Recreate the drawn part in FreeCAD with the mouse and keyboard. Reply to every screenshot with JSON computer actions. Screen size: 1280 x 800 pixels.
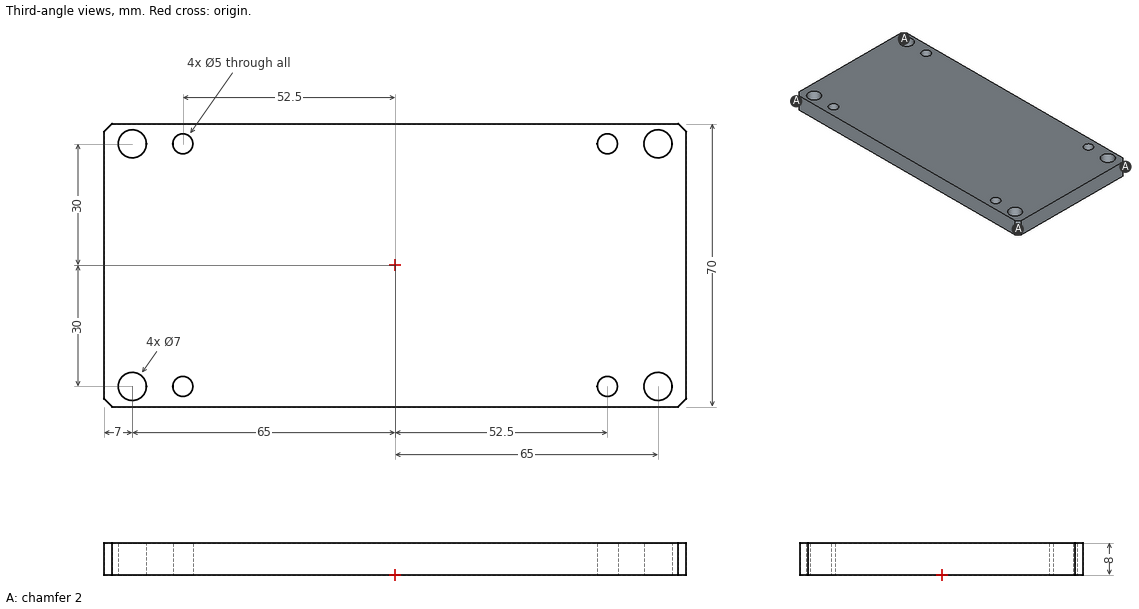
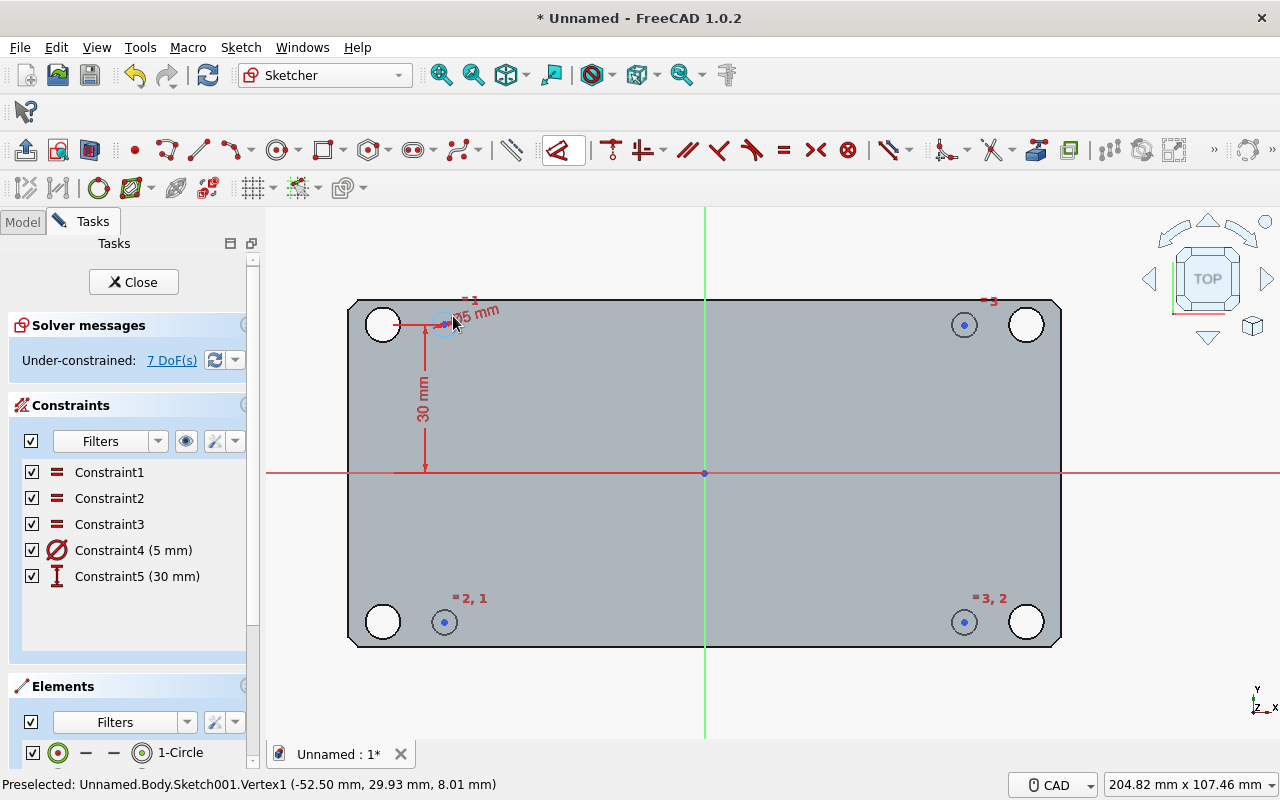
{"action": "left_click", "coordinate": [445, 622]}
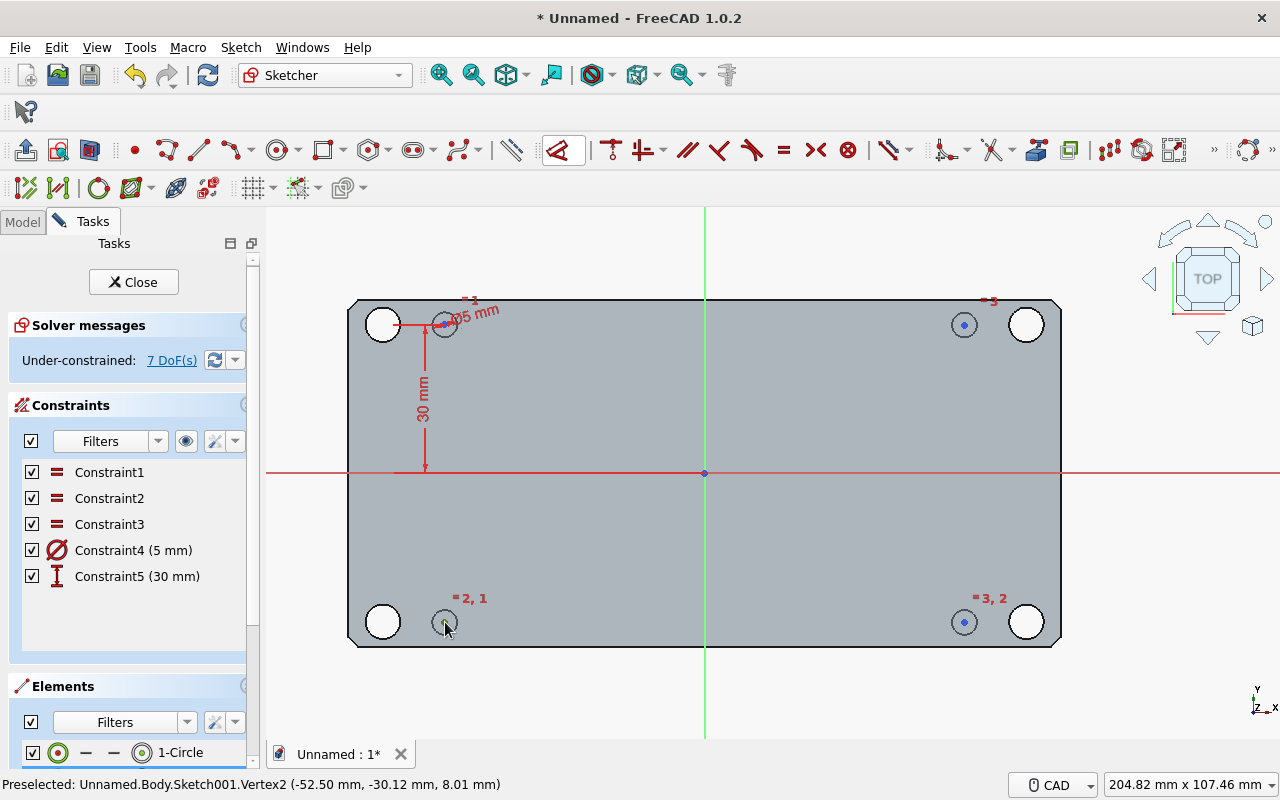
{"action": "key", "text": "i"}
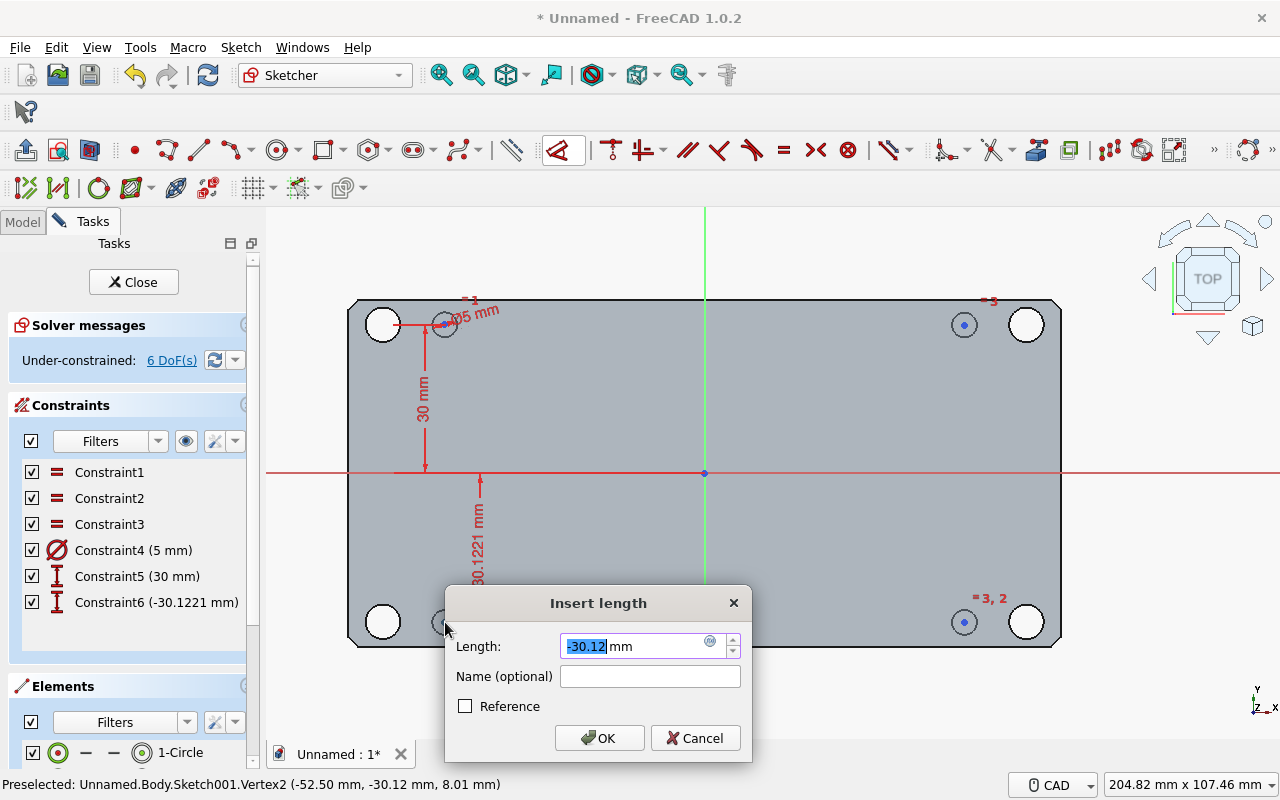
{"action": "type", "text": "-30"}
{"action": "key", "text": "Return"}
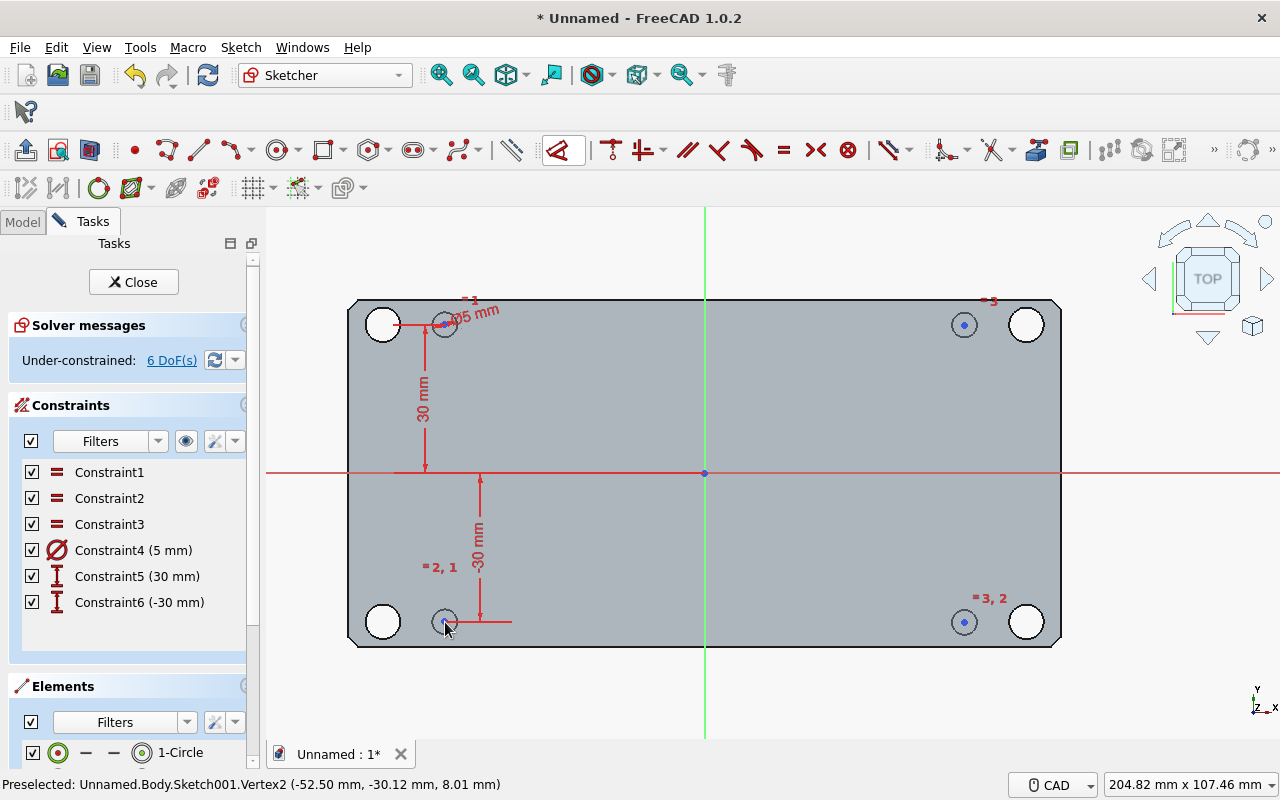
{"action": "left_click", "coordinate": [964, 622]}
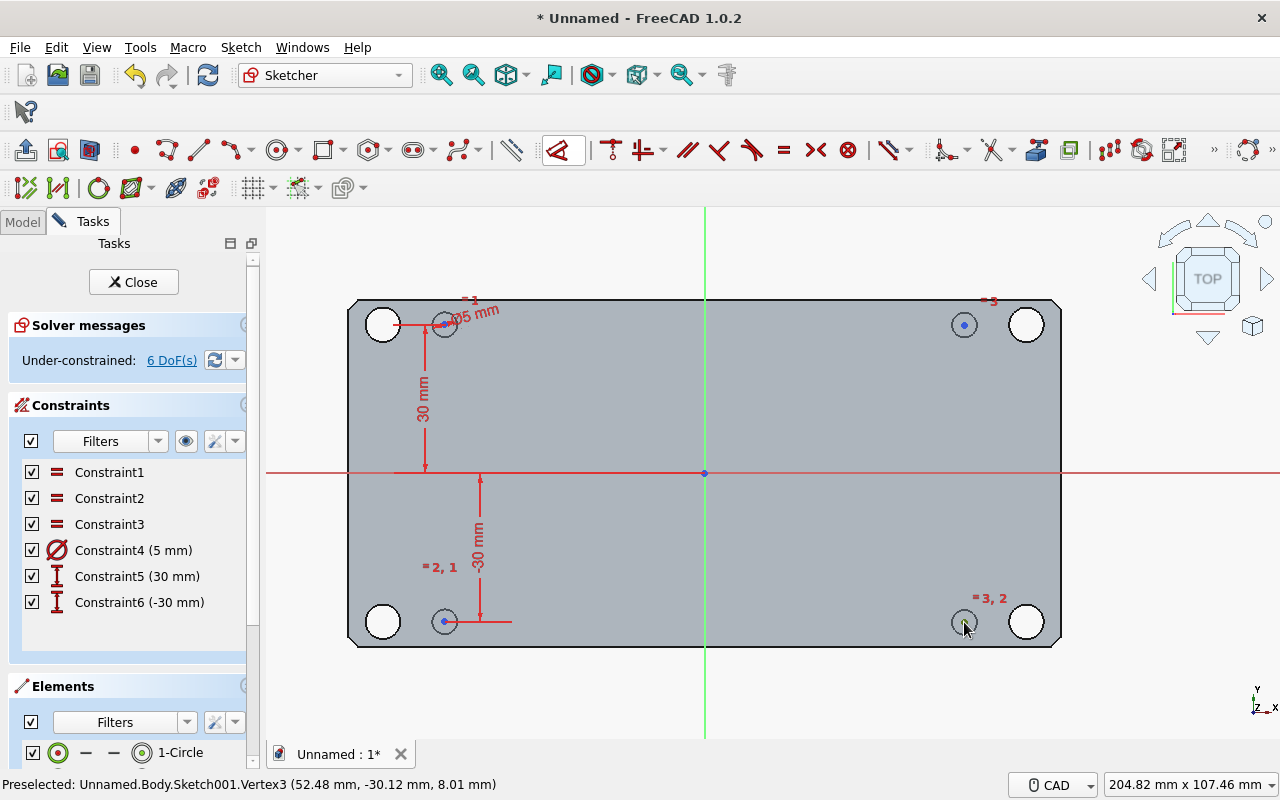
{"action": "left_click", "coordinate": [580, 150]}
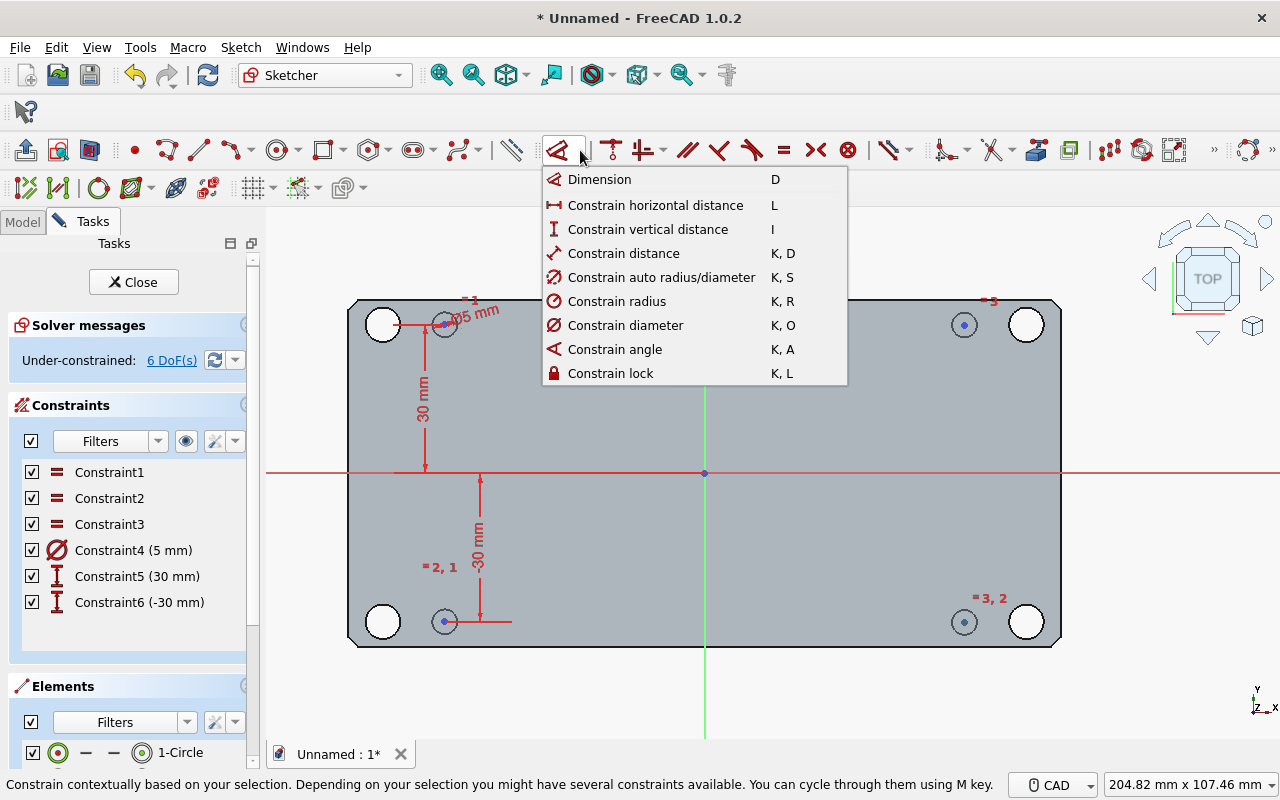
{"action": "left_click", "coordinate": [695, 229]}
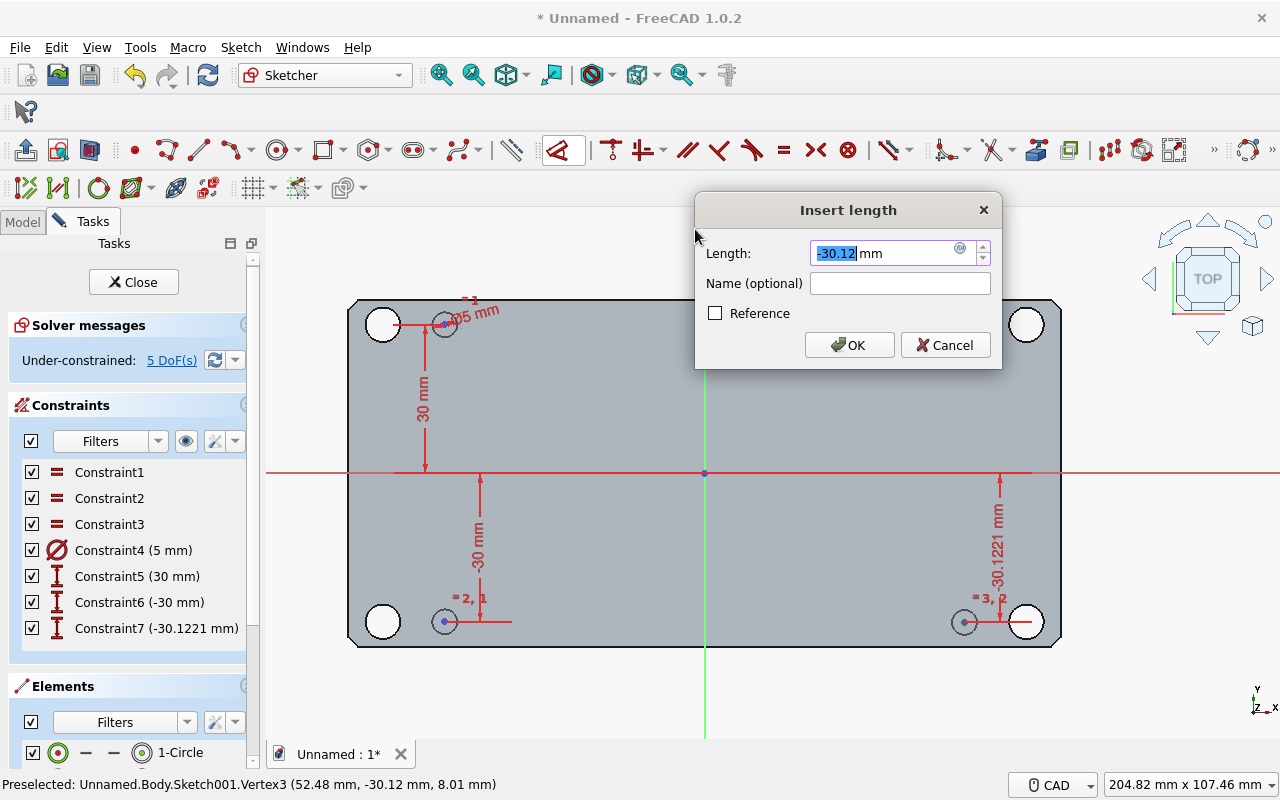
{"action": "type", "text": "-30"}
{"action": "key", "text": "Return"}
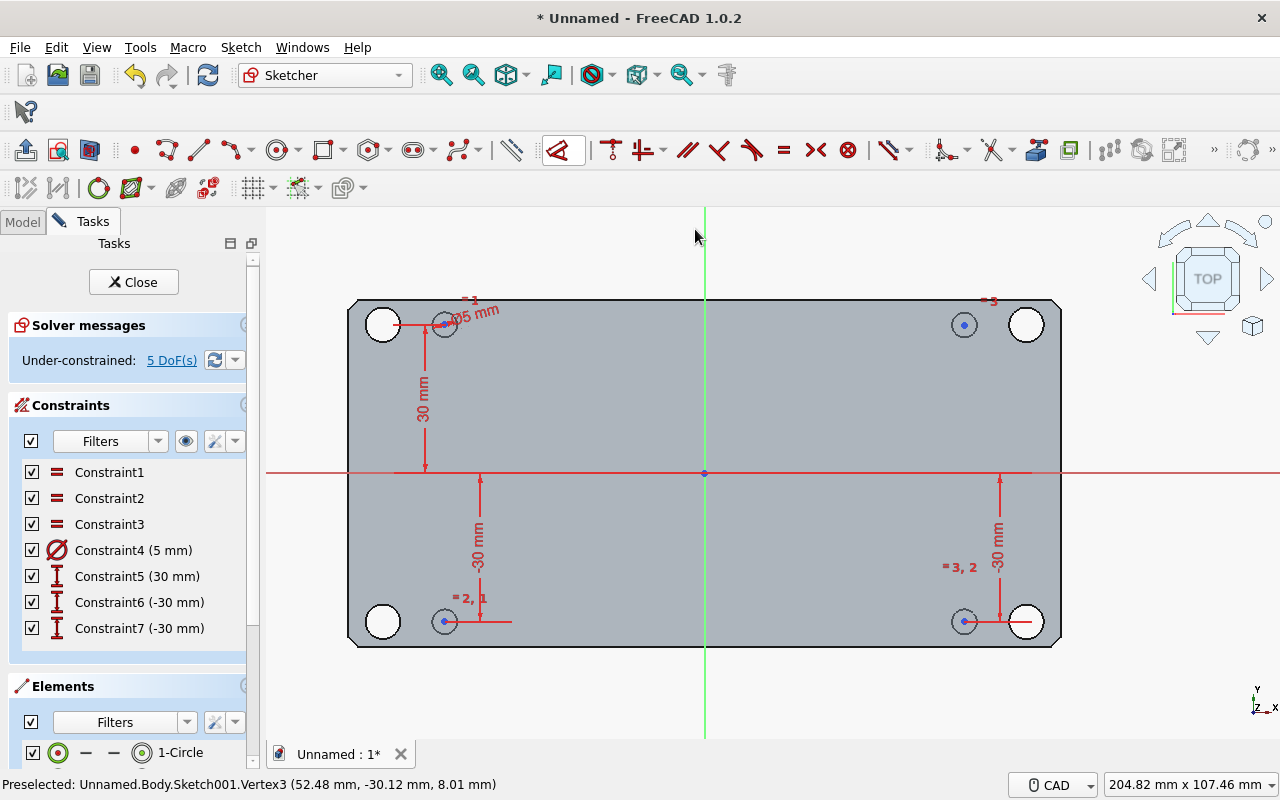
{"action": "left_click", "coordinate": [964, 325]}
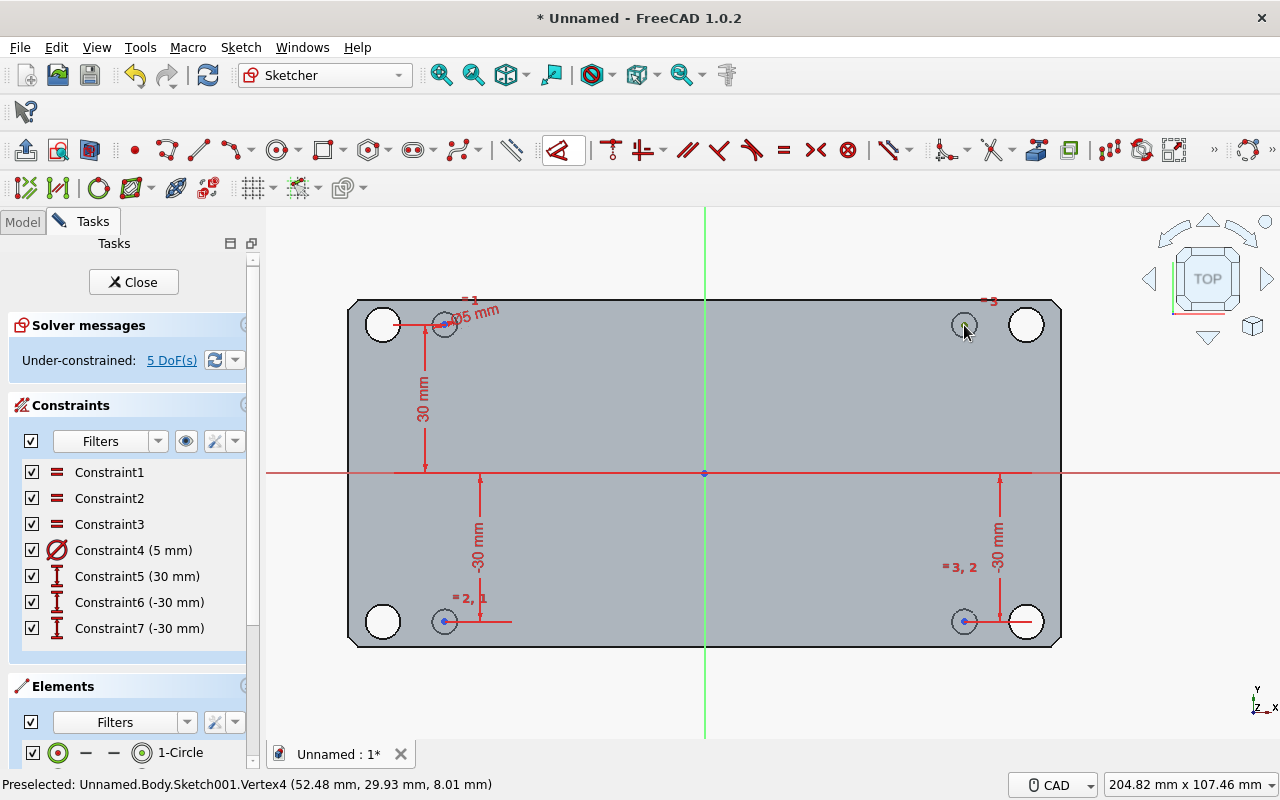
{"action": "left_click", "coordinate": [580, 150]}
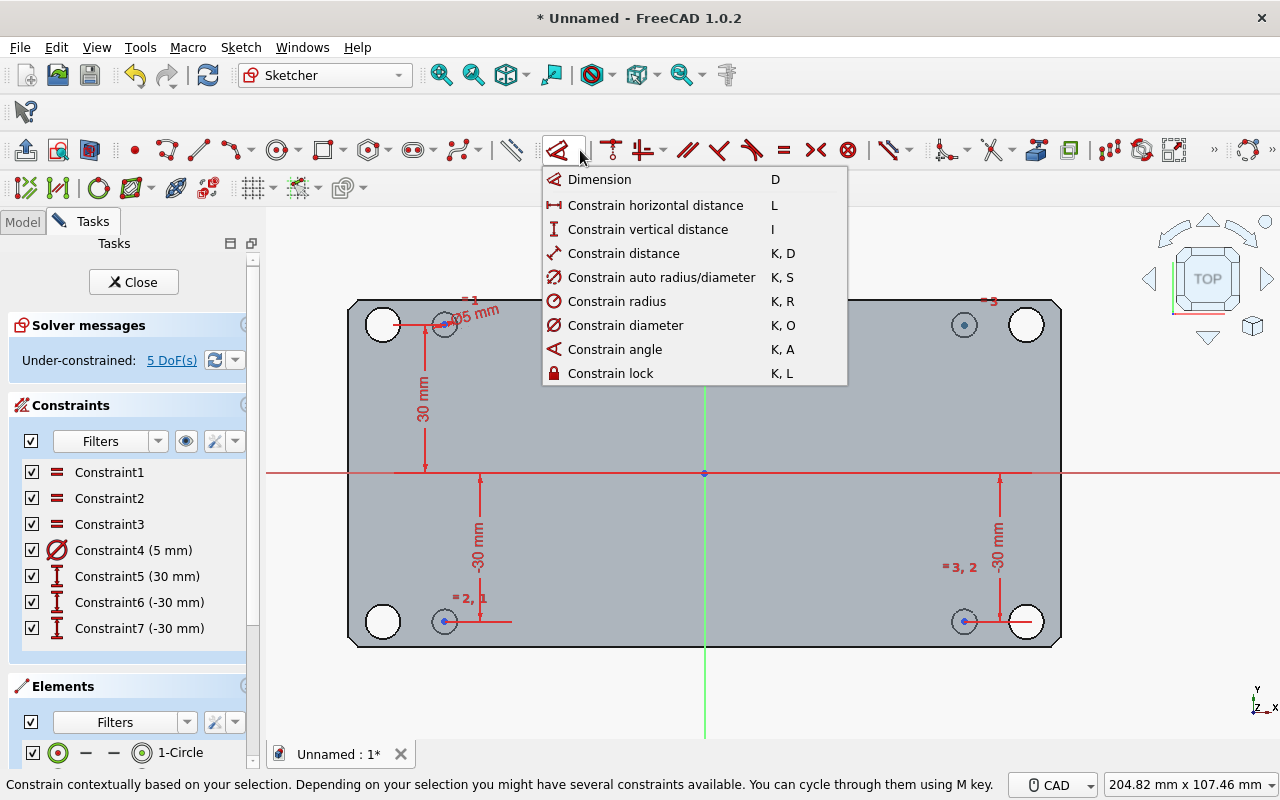
{"action": "left_click", "coordinate": [695, 229]}